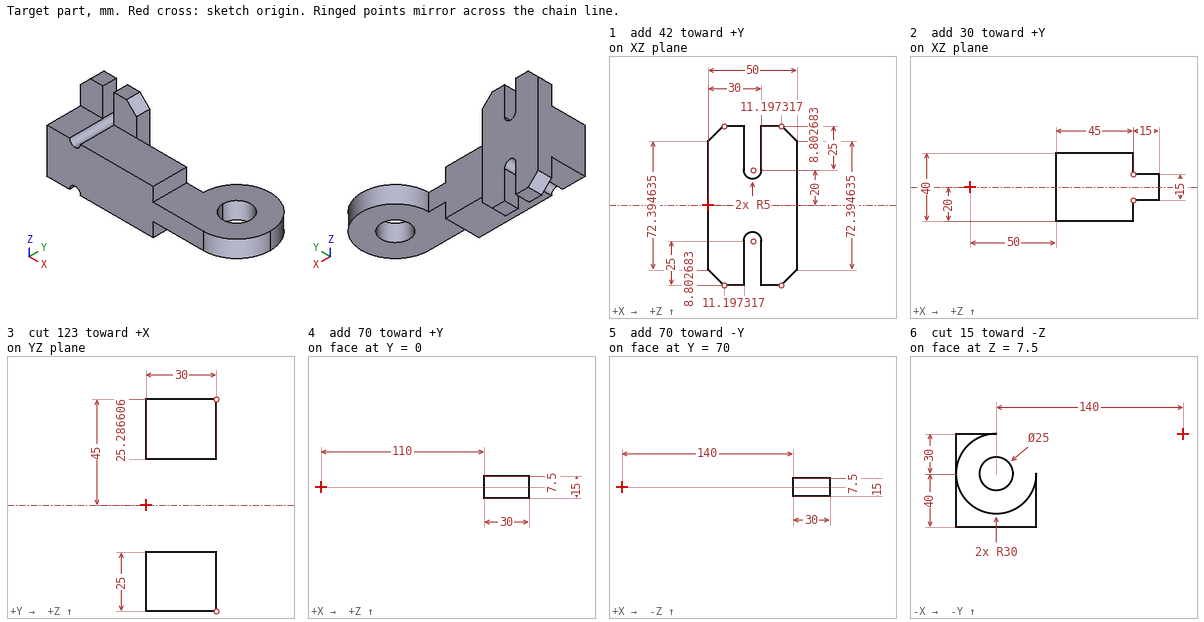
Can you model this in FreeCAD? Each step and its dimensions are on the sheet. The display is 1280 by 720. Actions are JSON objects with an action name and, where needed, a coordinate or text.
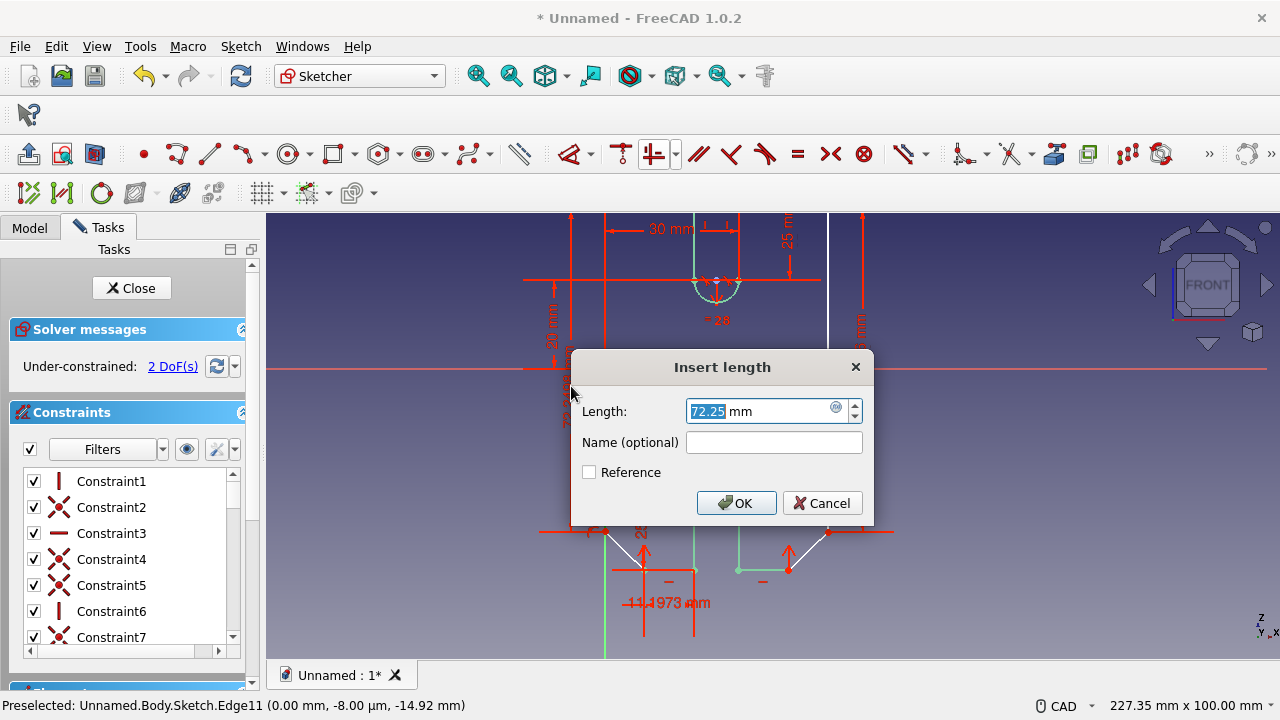
{"action": "type", "text": "72.394635"}
{"action": "key", "text": "Return"}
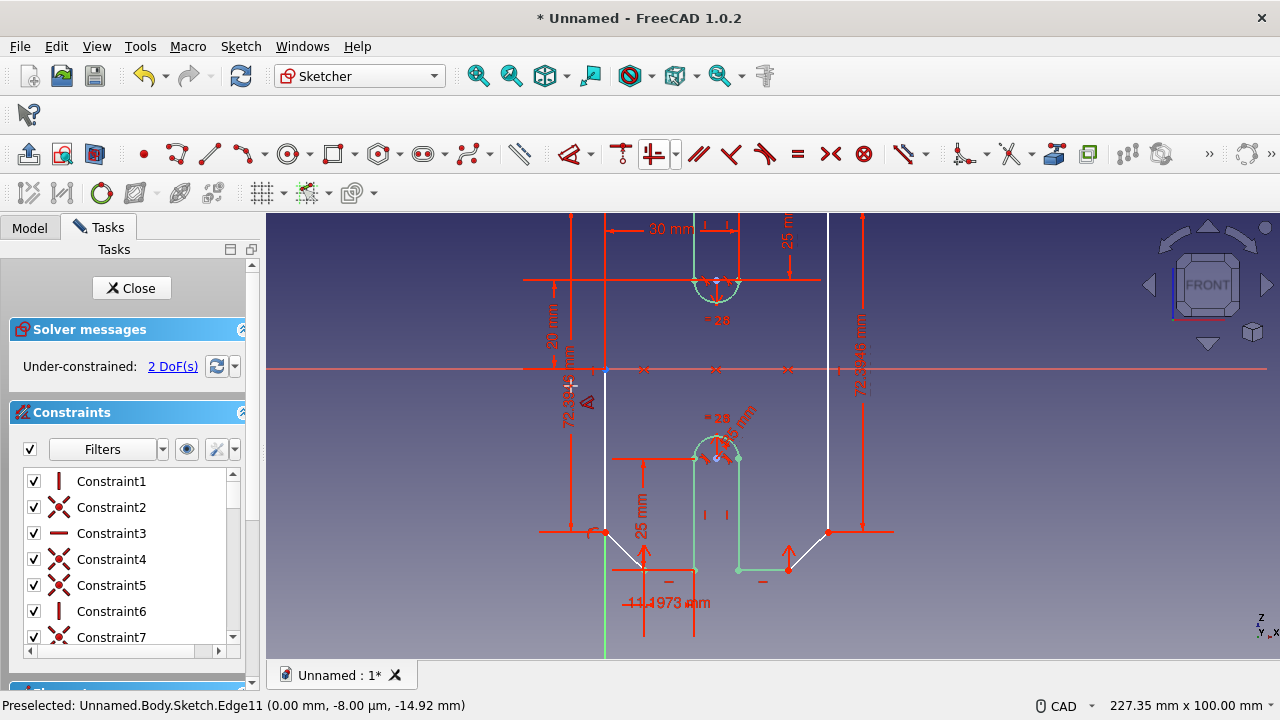
{"action": "scroll", "coordinate": [680, 571], "scroll_direction": "down", "scroll_amount": 2}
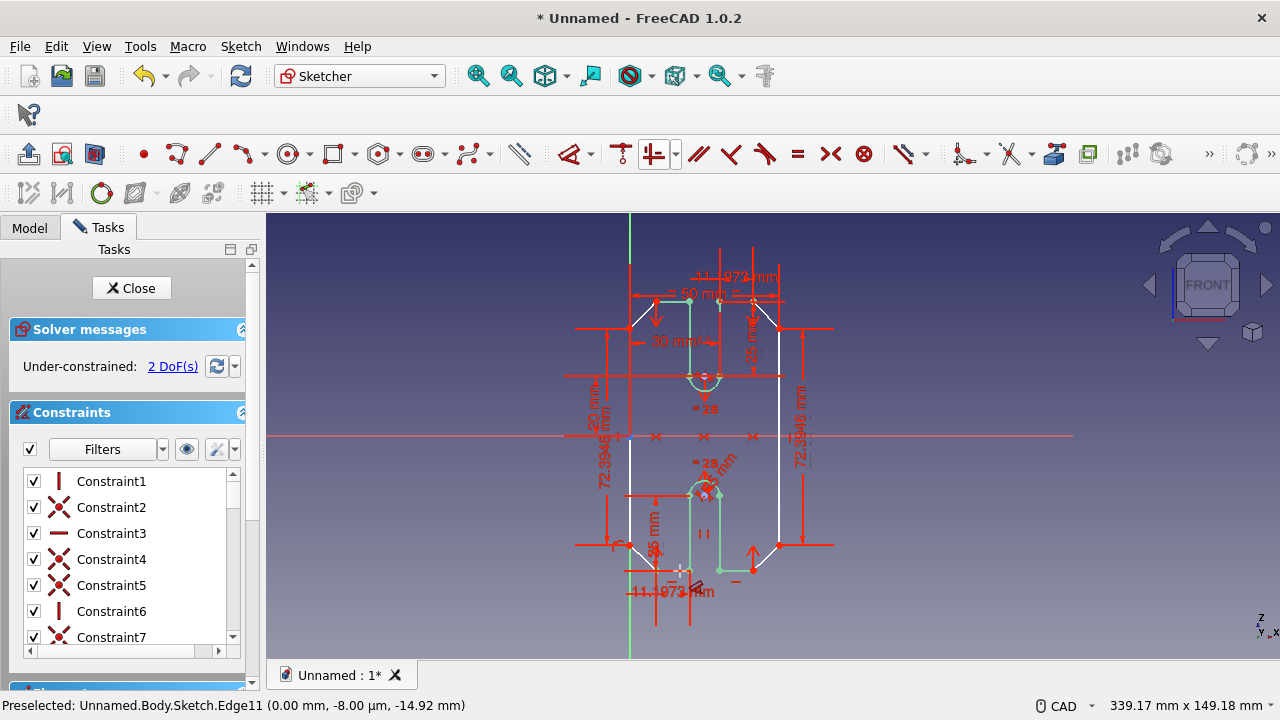
{"action": "scroll", "coordinate": [761, 310], "scroll_direction": "up", "scroll_amount": 3}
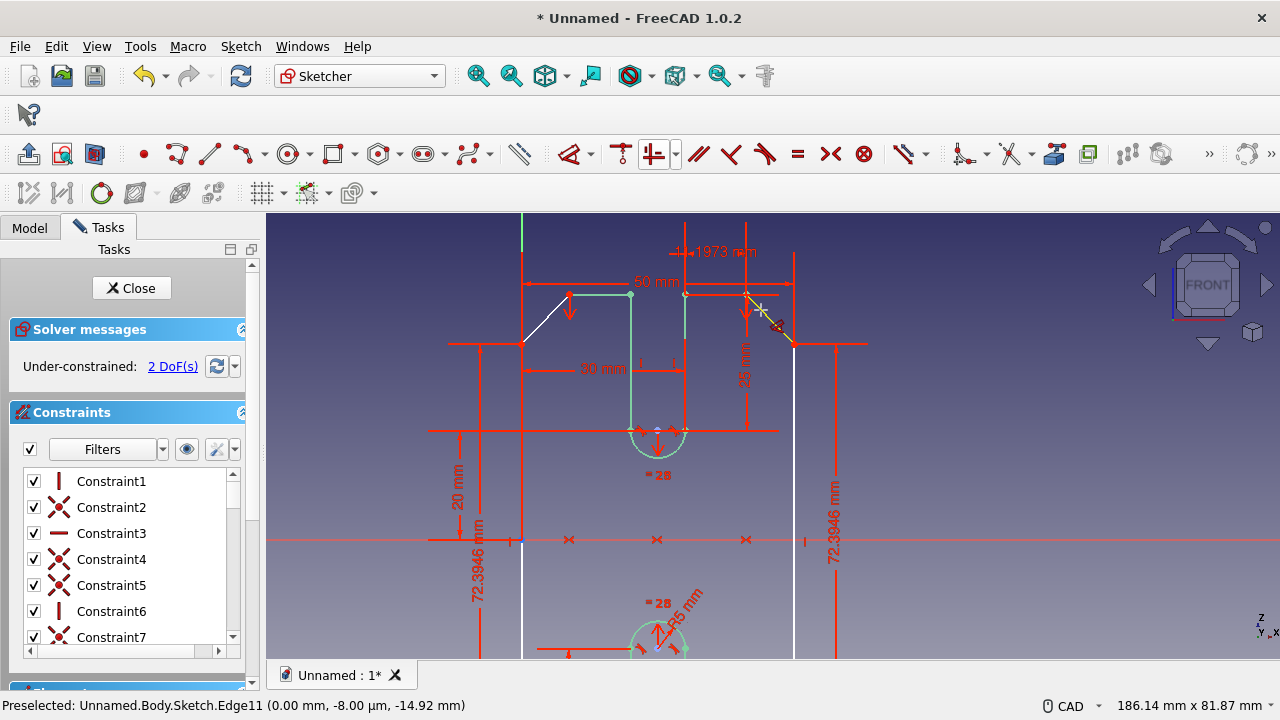
{"action": "left_click", "coordinate": [761, 309]}
{"action": "left_click", "coordinate": [828, 319]}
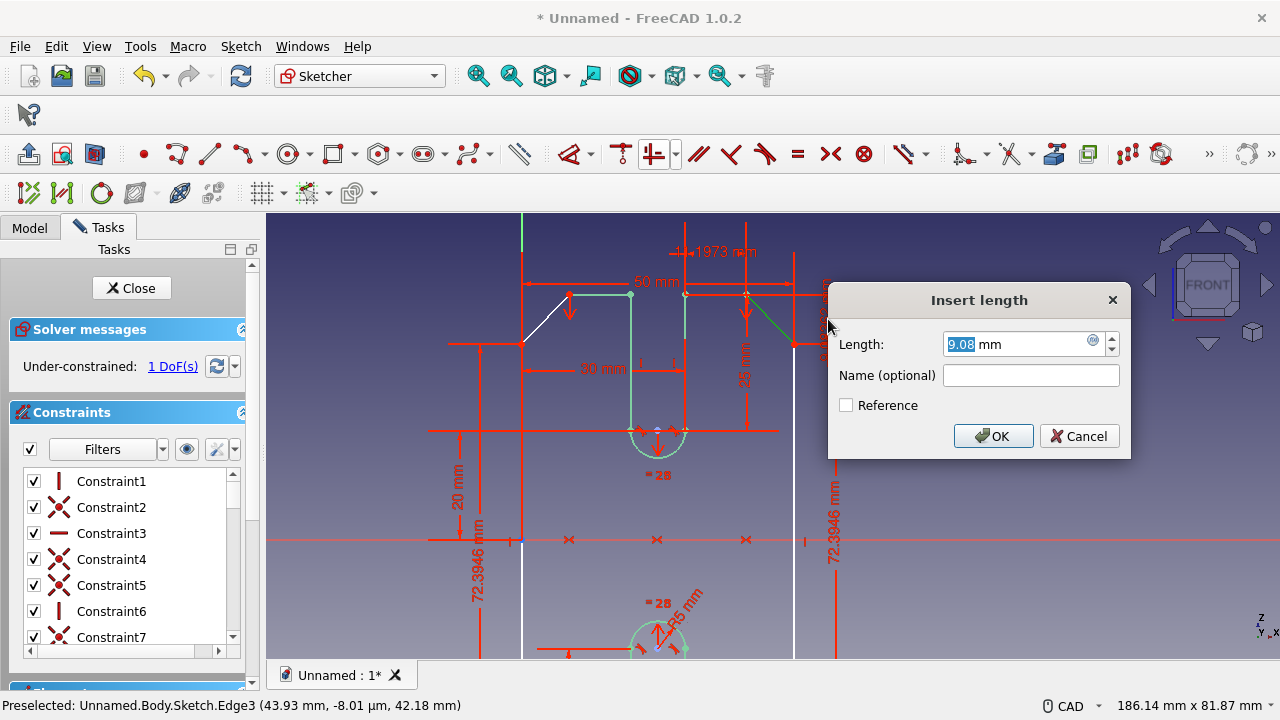
{"action": "type", "text": "8.802683"}
{"action": "key", "text": "Return"}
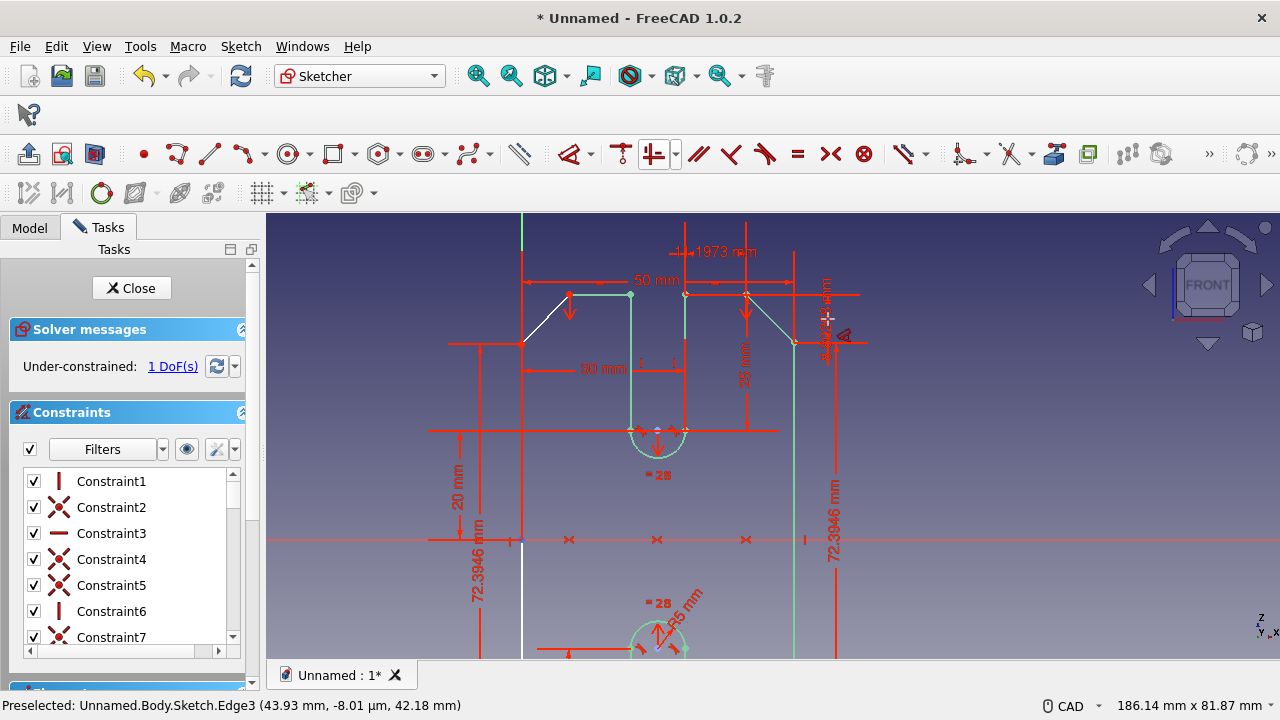
{"action": "scroll", "coordinate": [761, 310], "scroll_direction": "down", "scroll_amount": 3}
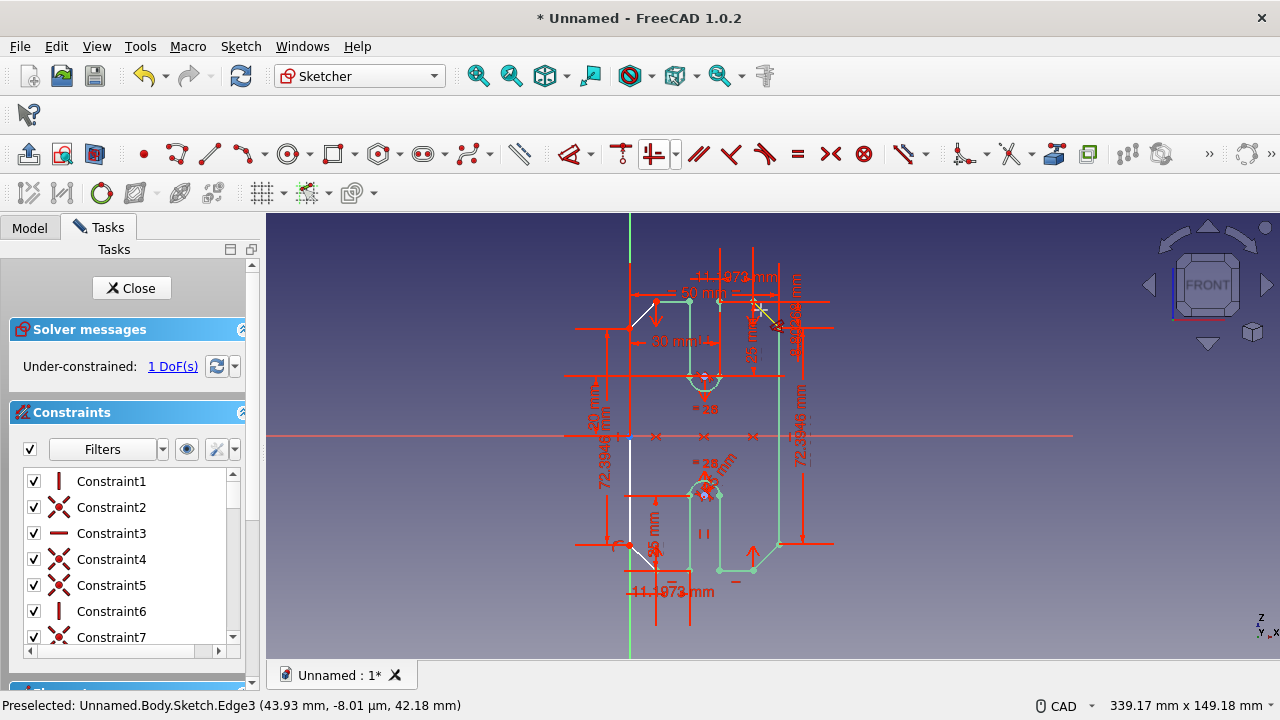
{"action": "scroll", "coordinate": [648, 563], "scroll_direction": "up", "scroll_amount": 3}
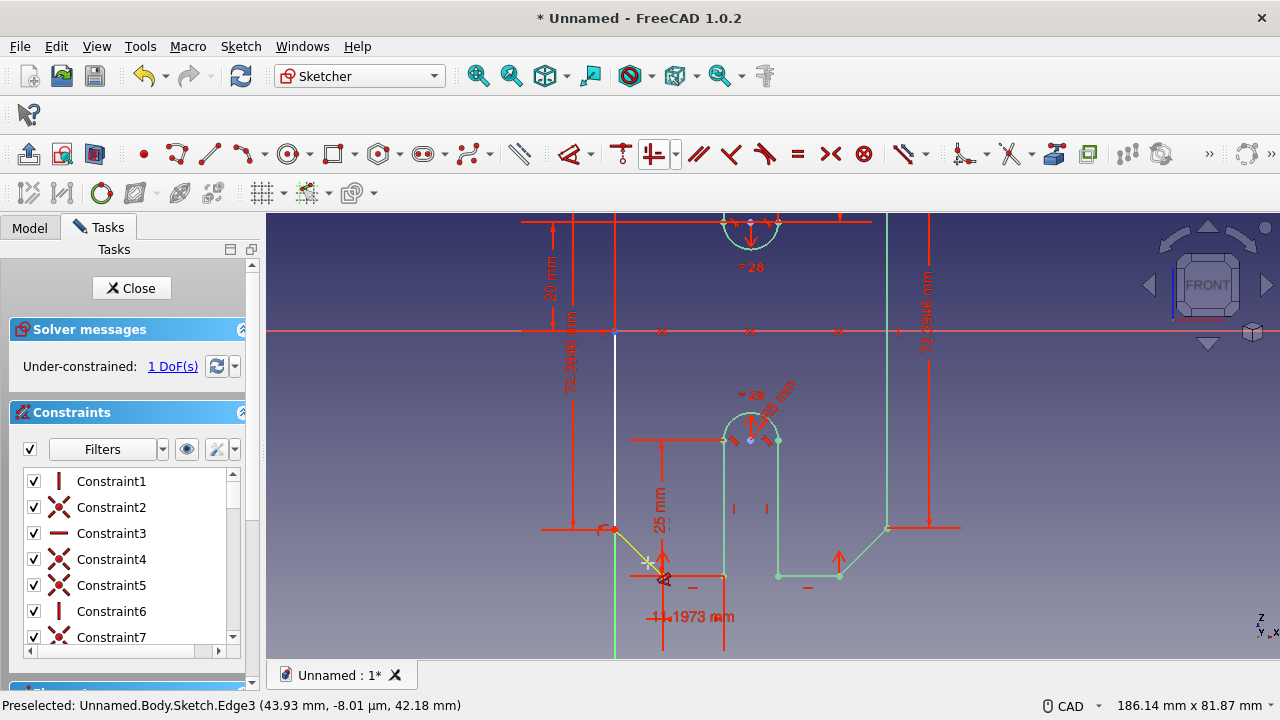
{"action": "left_click", "coordinate": [648, 562]}
{"action": "left_click", "coordinate": [581, 553]}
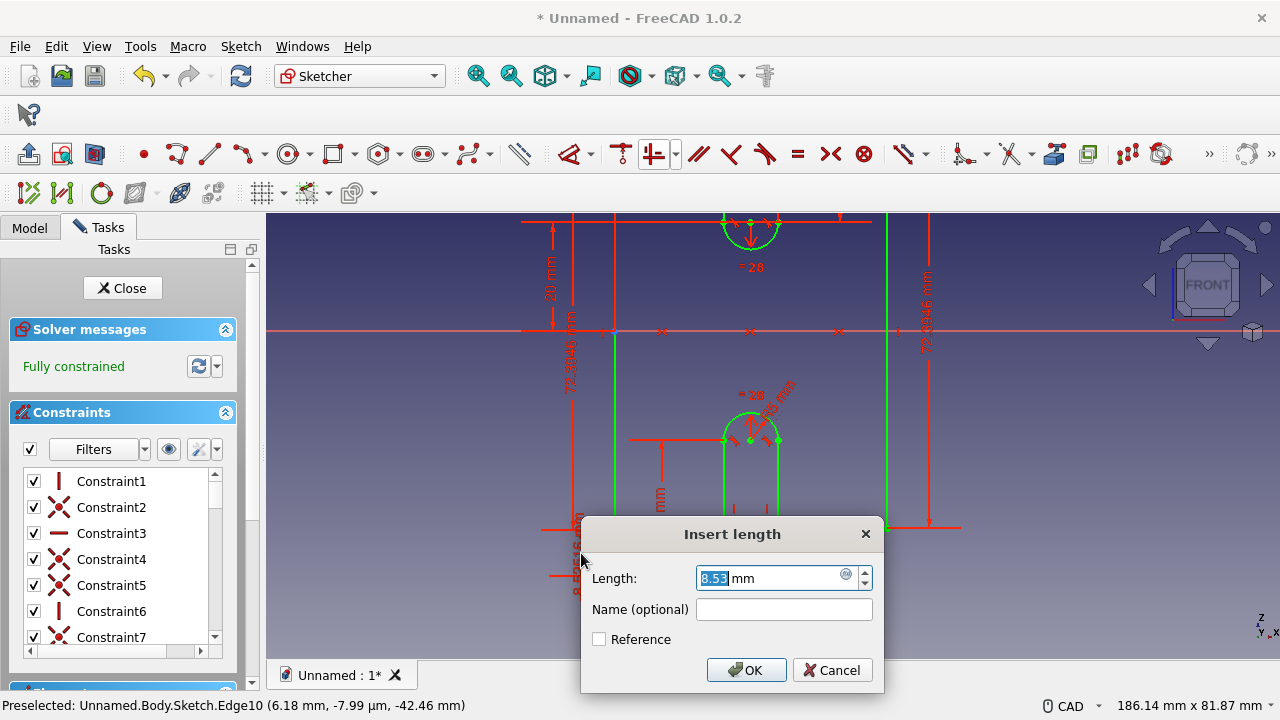
{"action": "type", "text": "8.802683"}
{"action": "key", "text": "Return"}
{"action": "key", "text": "Escape"}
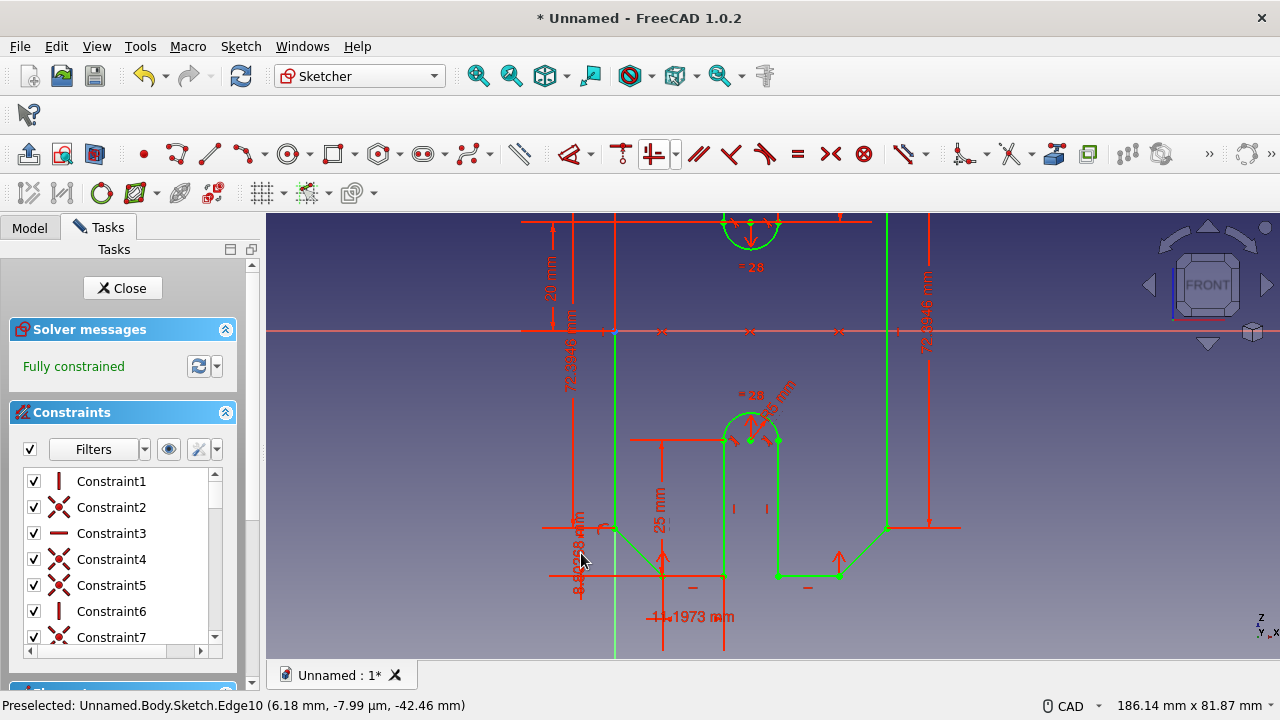
{"action": "left_click", "coordinate": [123, 288]}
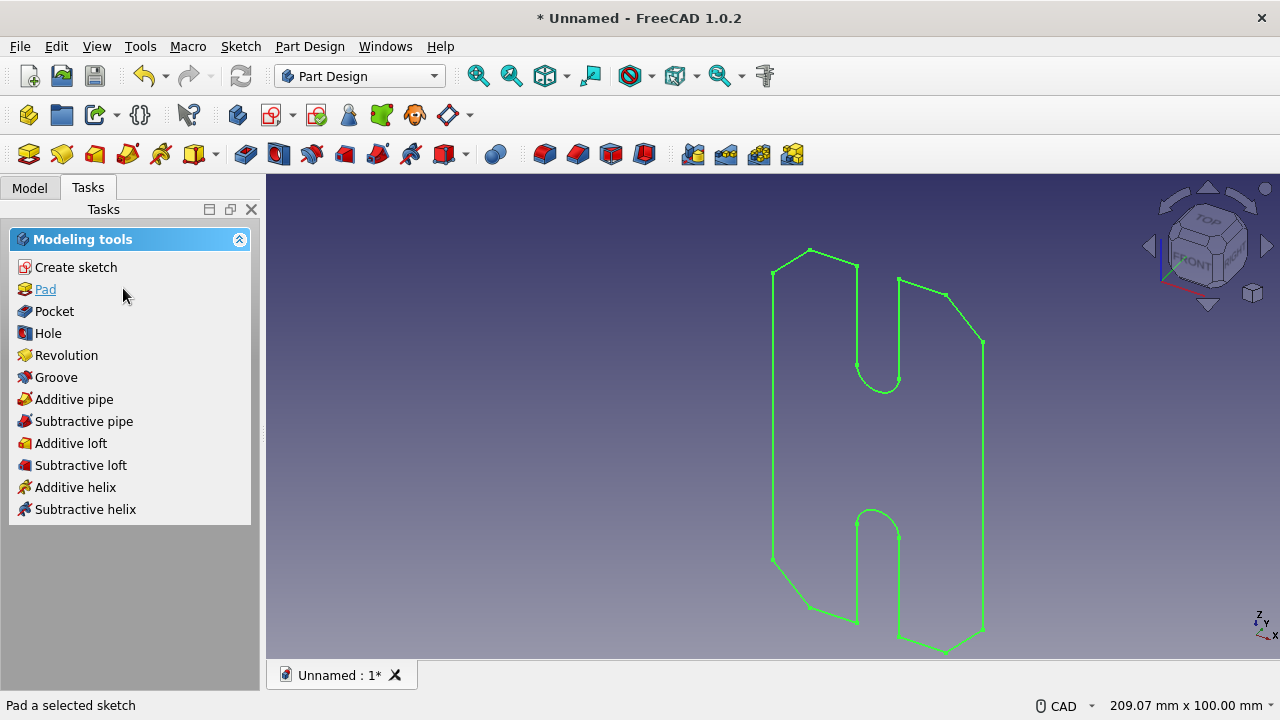
{"action": "left_click", "coordinate": [29, 154]}